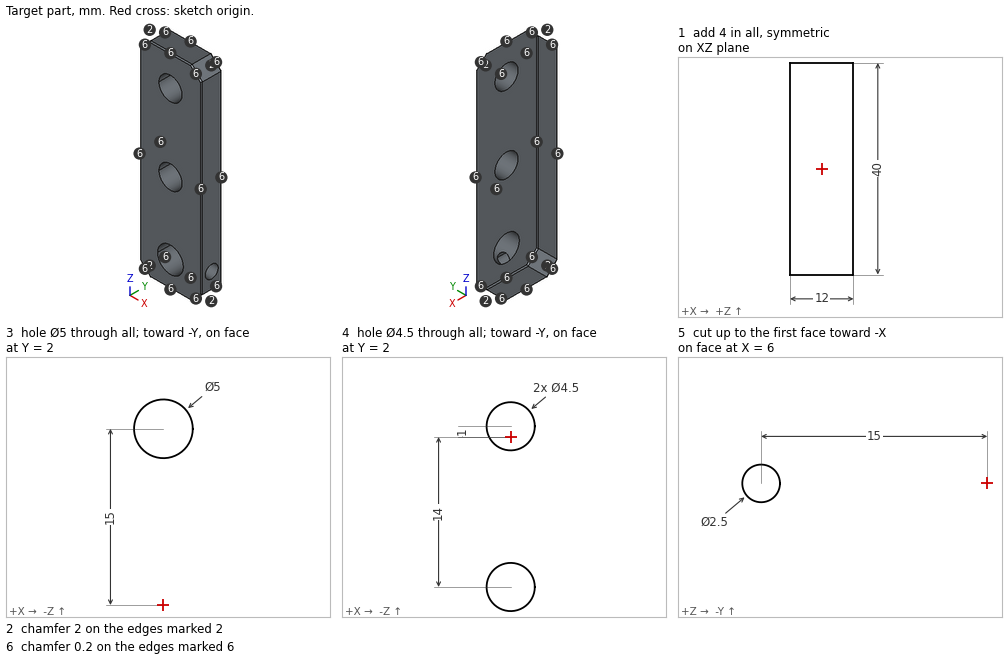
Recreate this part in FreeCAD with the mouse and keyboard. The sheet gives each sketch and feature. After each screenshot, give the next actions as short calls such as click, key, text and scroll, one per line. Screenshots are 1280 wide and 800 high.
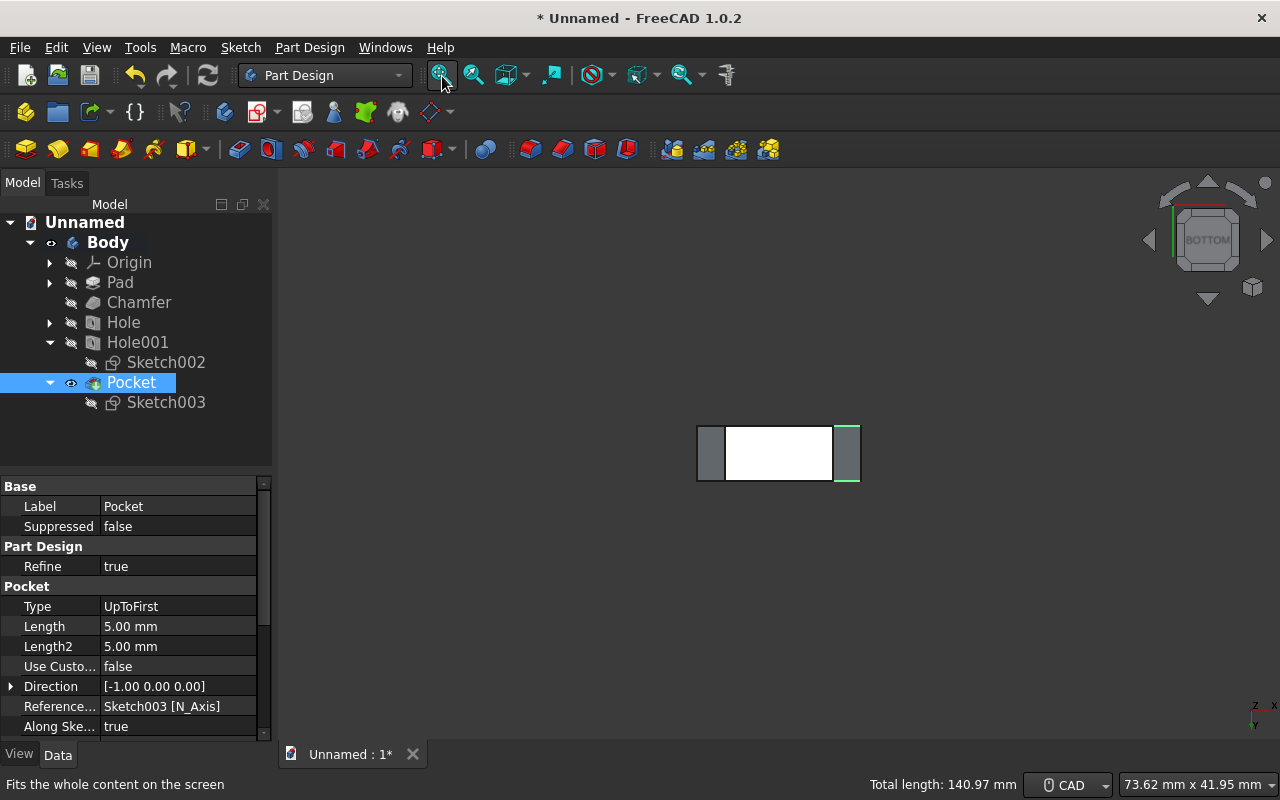
click(779, 425, ctrl)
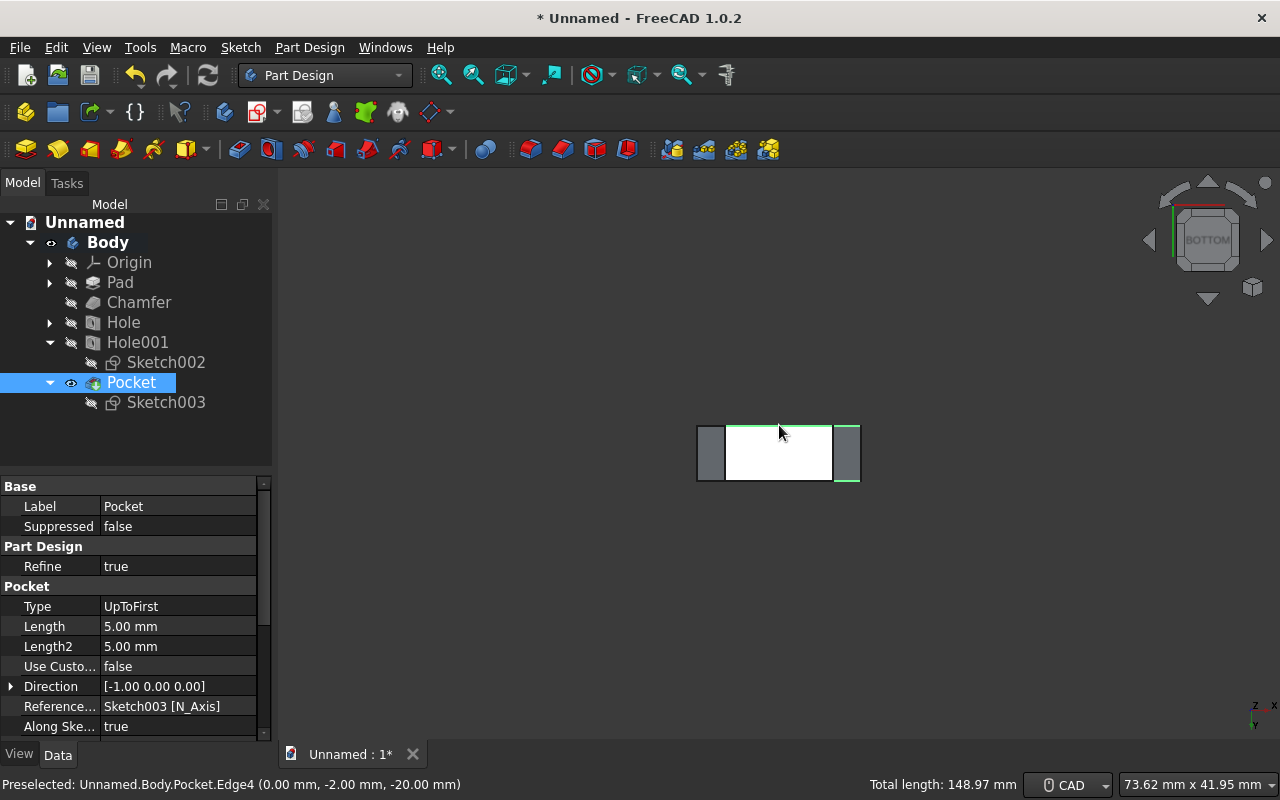
click(711, 425, ctrl)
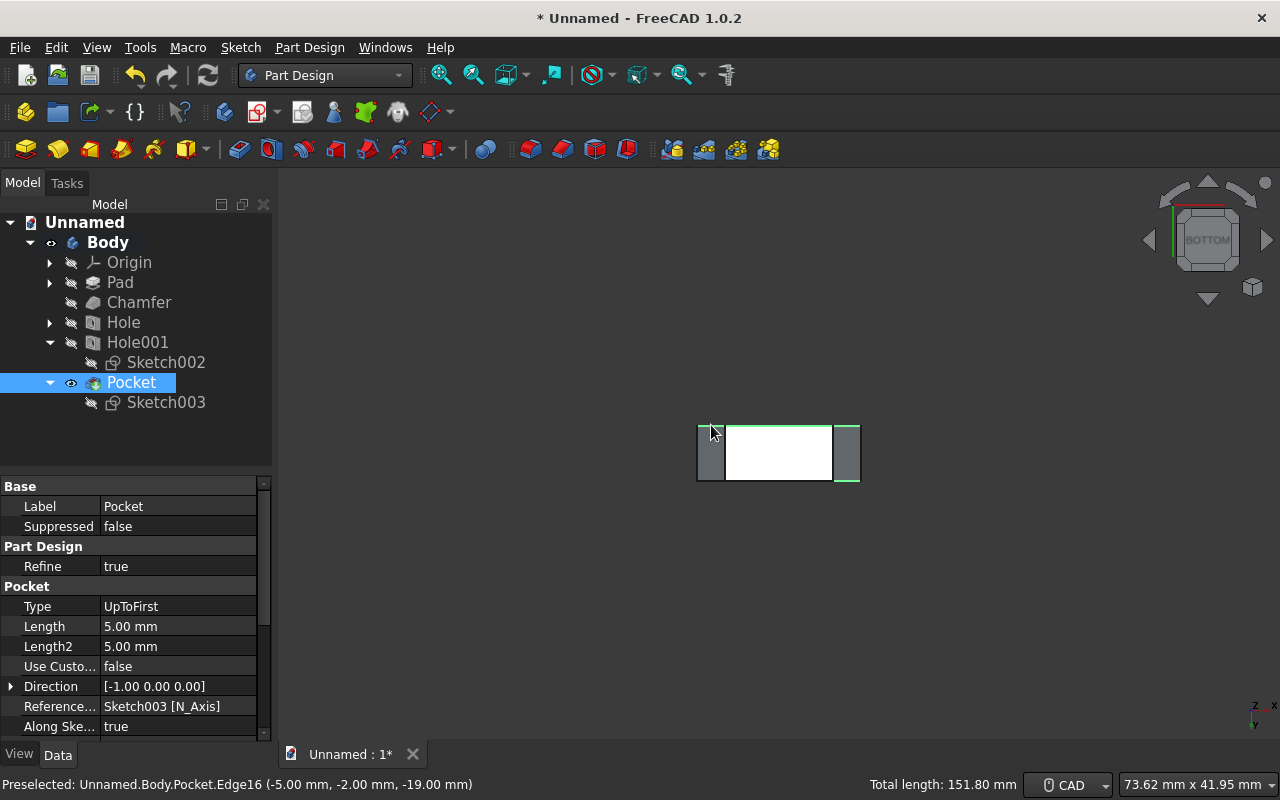
key(4)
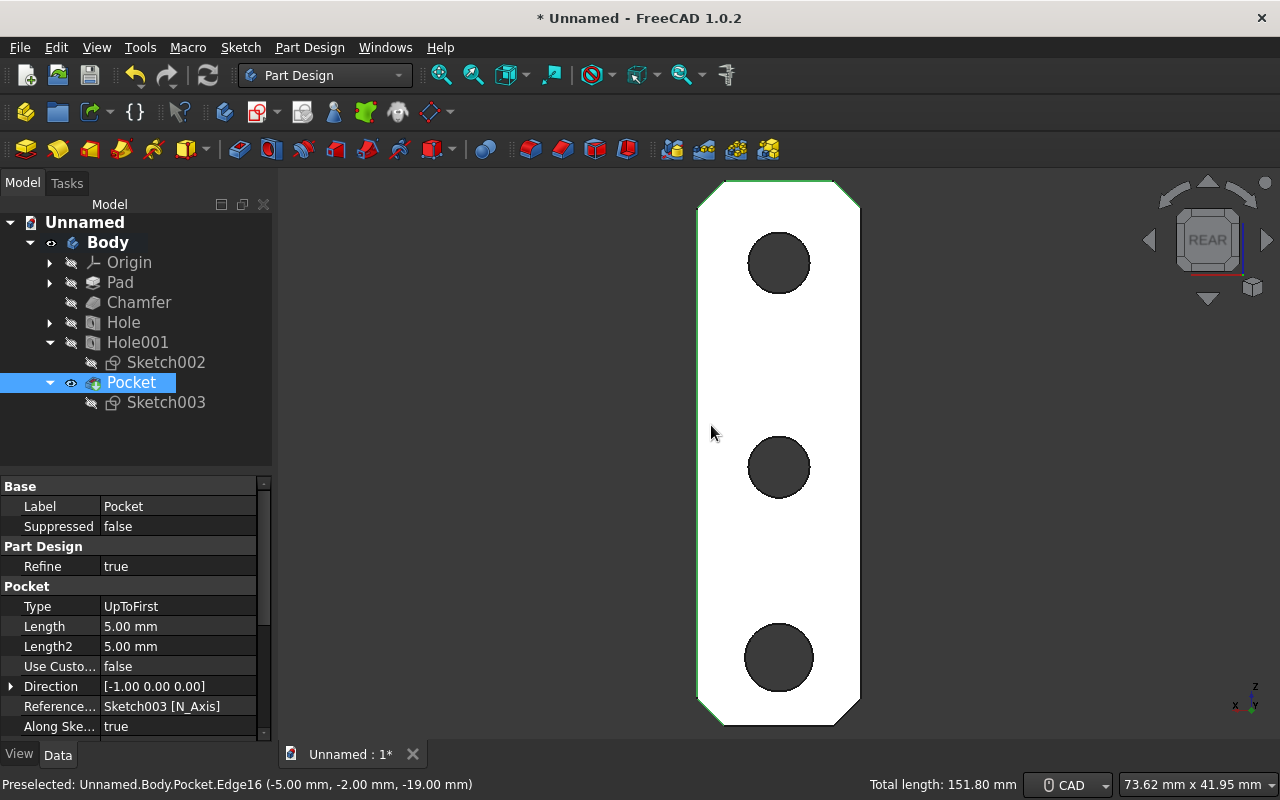
click(861, 452, ctrl)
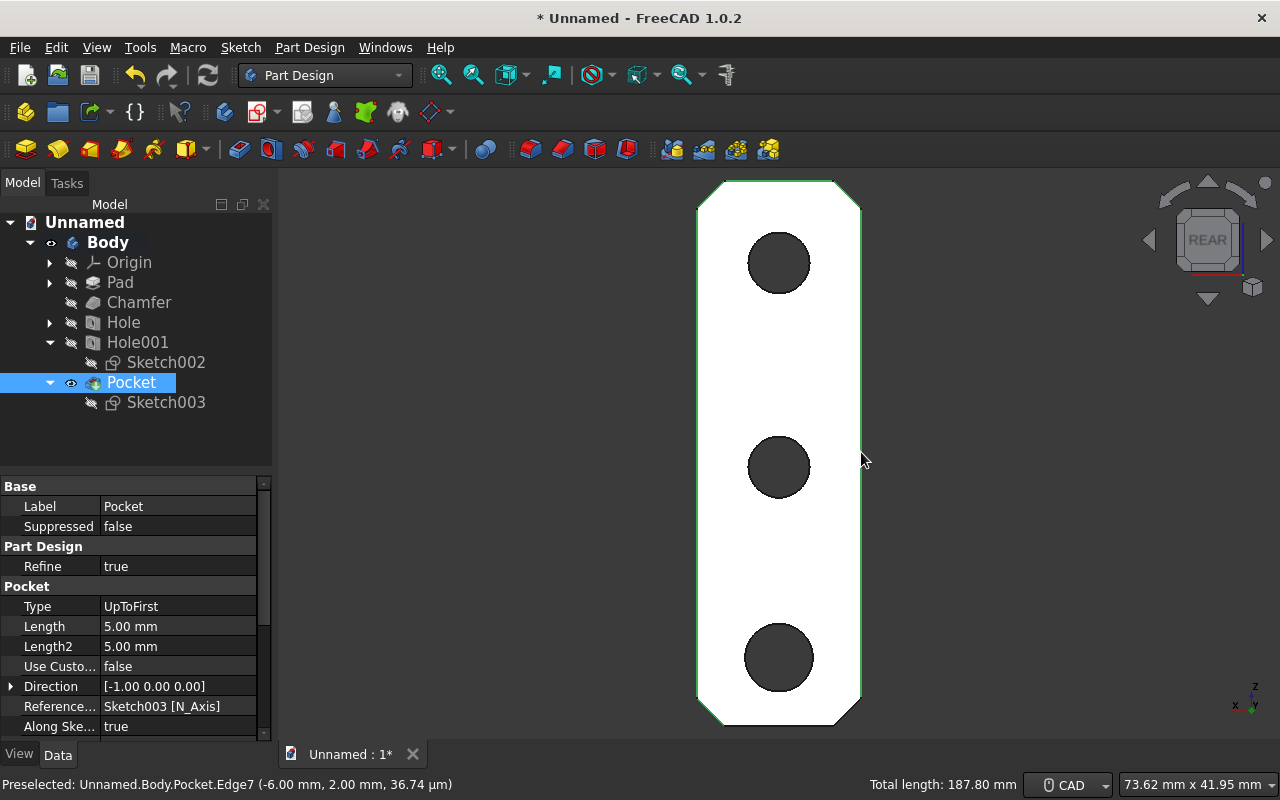
click(850, 708, ctrl)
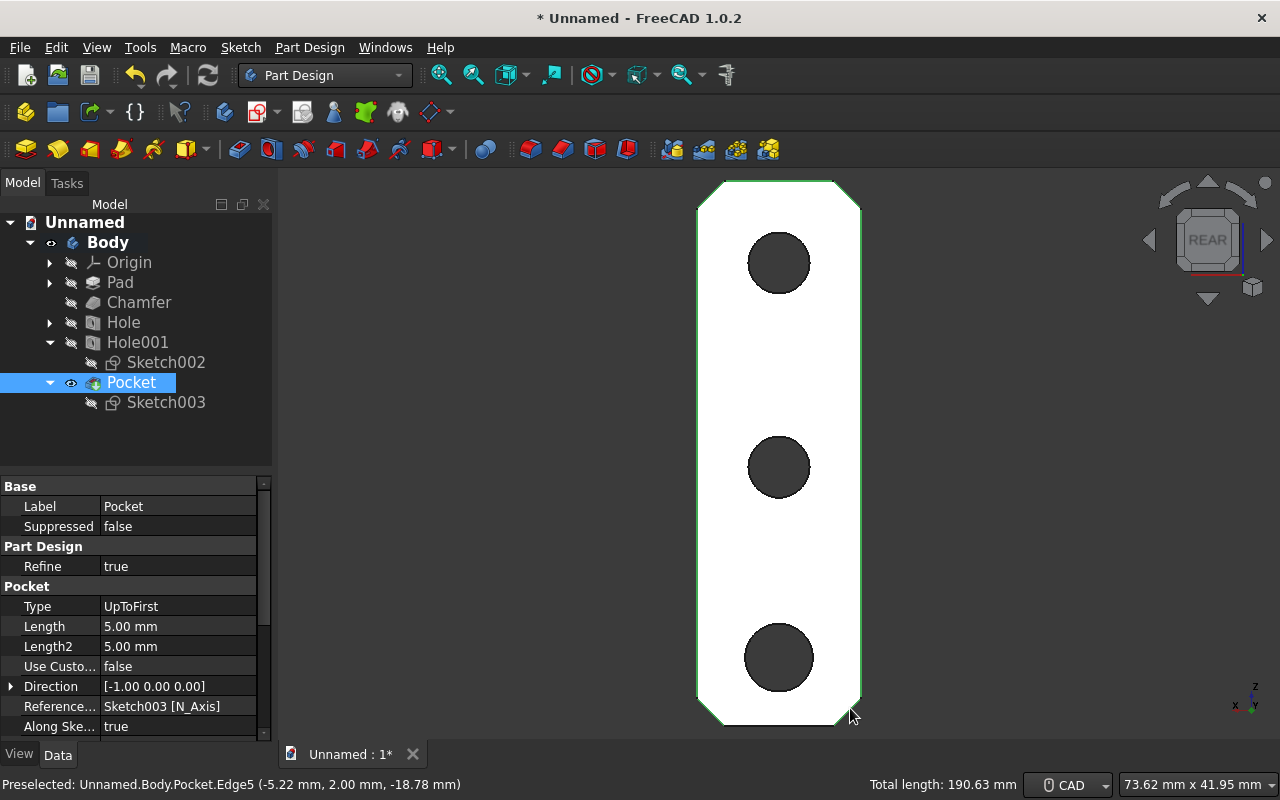
key(6)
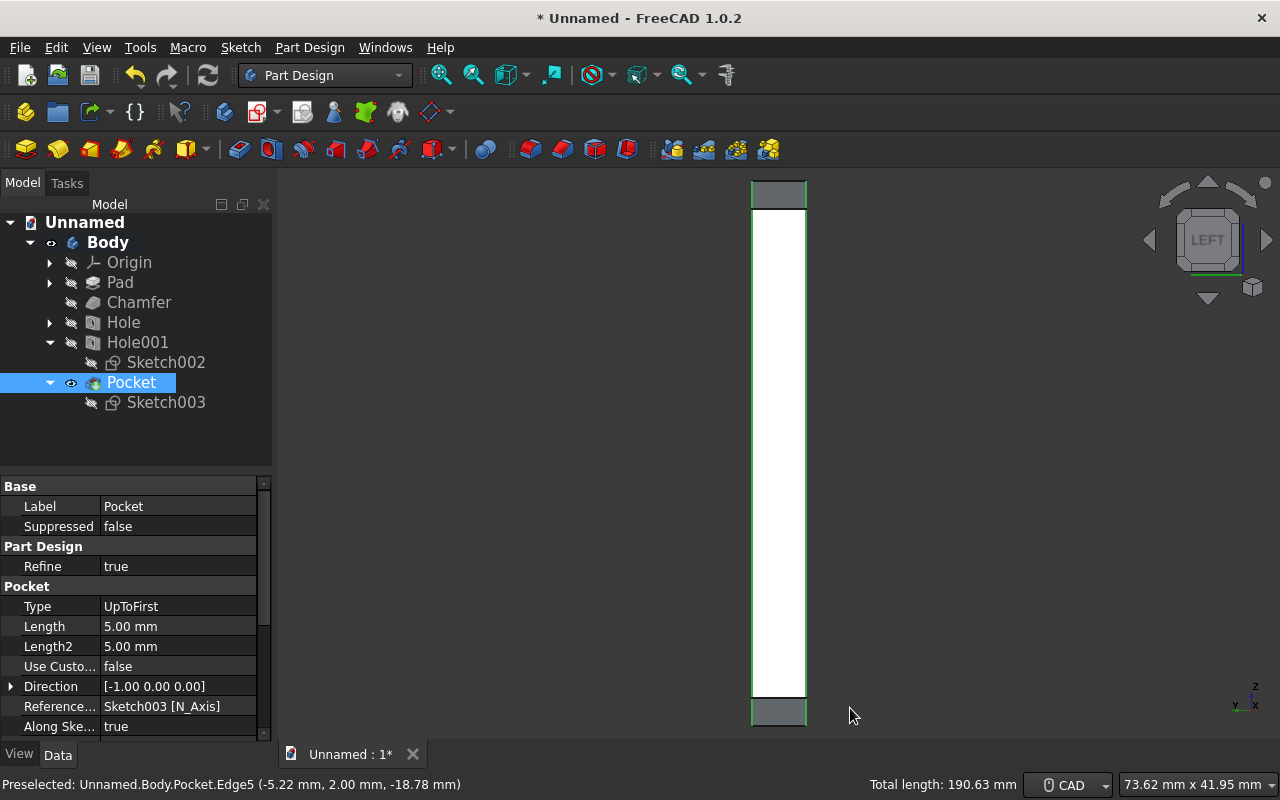
key(v)
key(3)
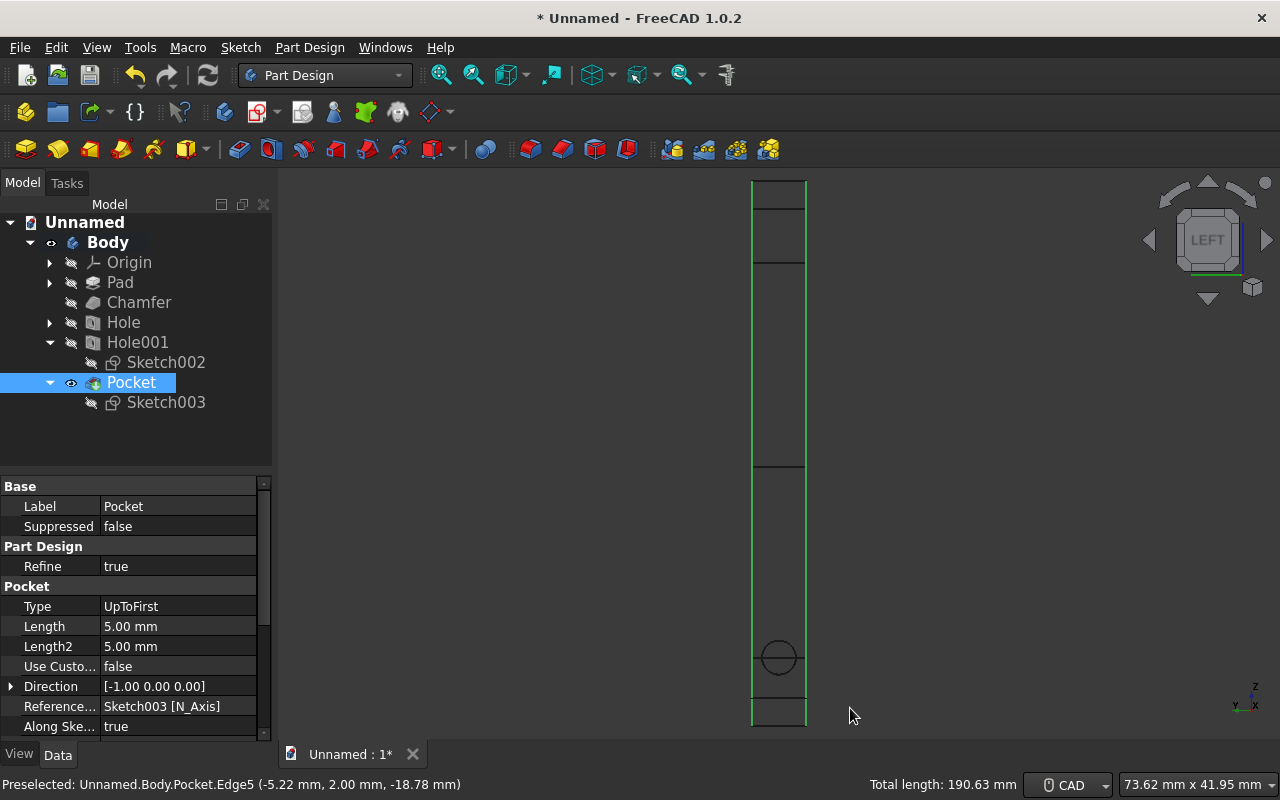
key(0)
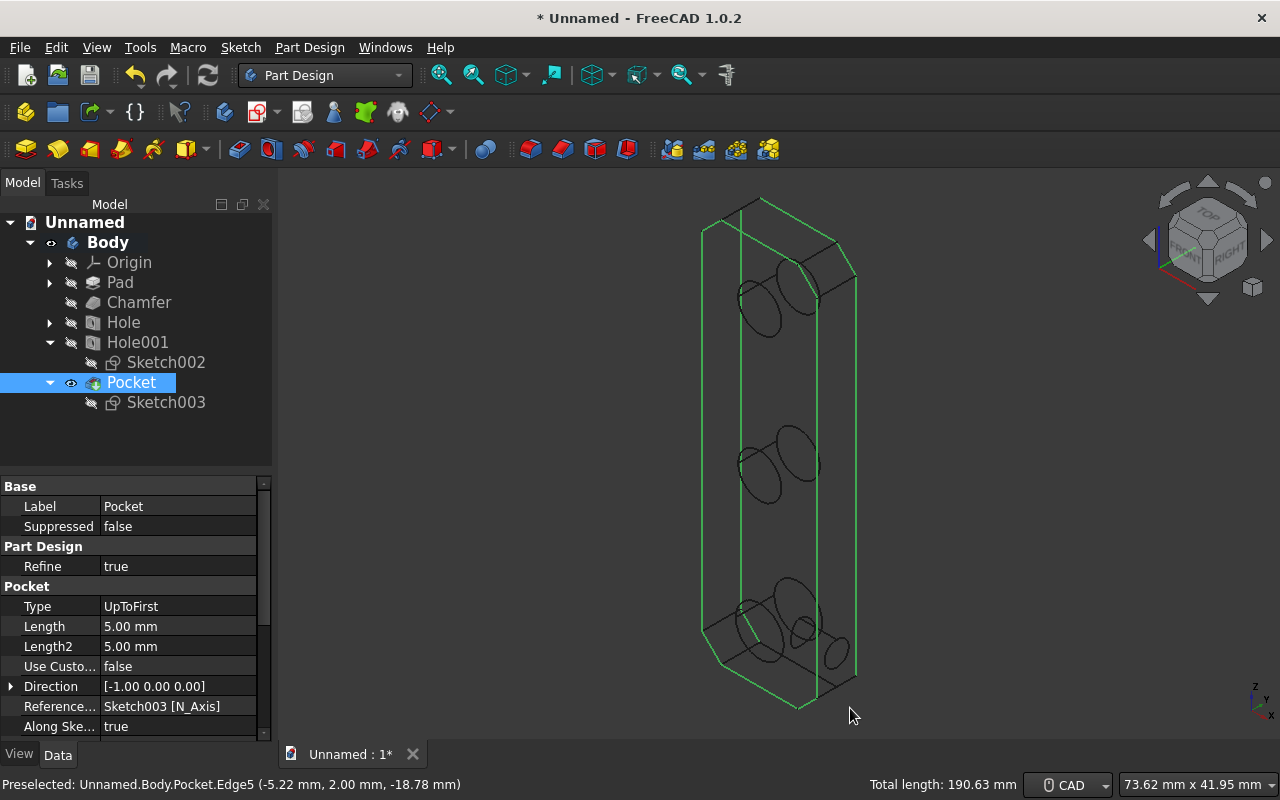
click(798, 664, ctrl)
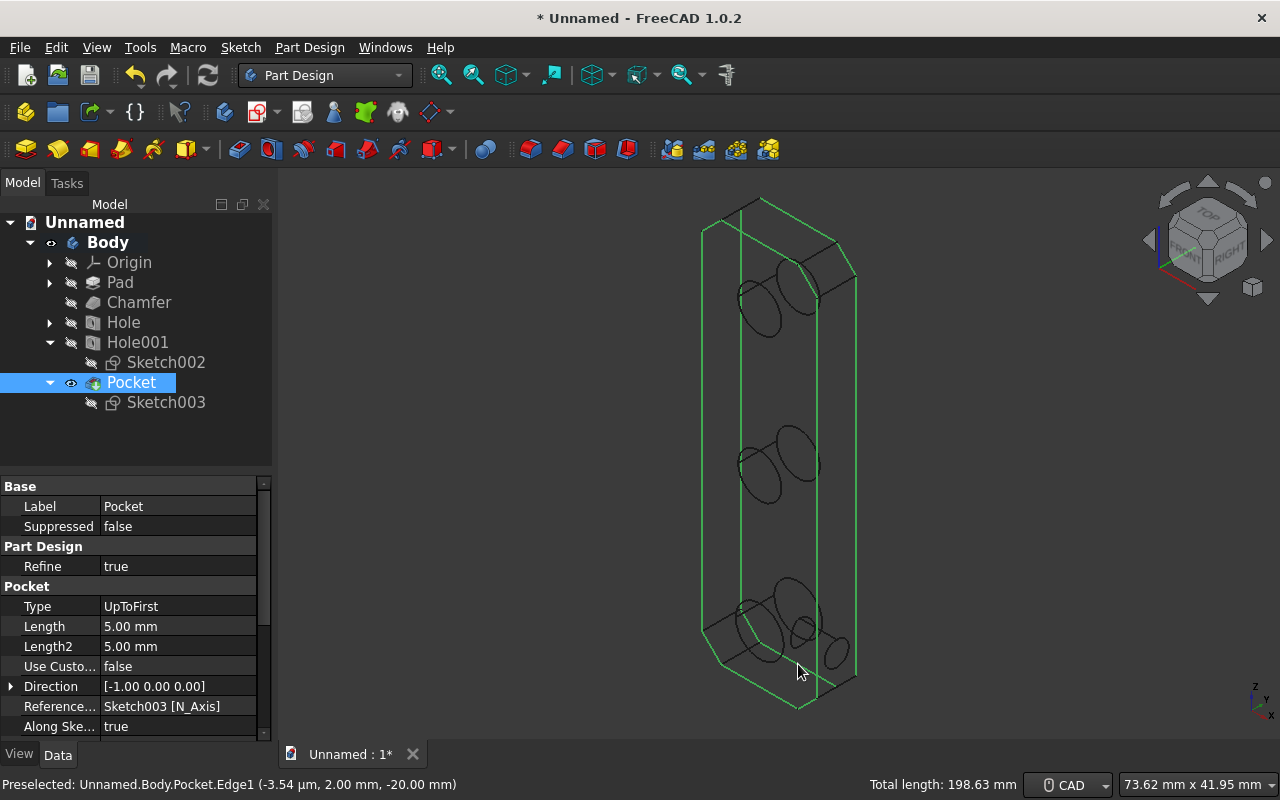
key(v)
key(1)